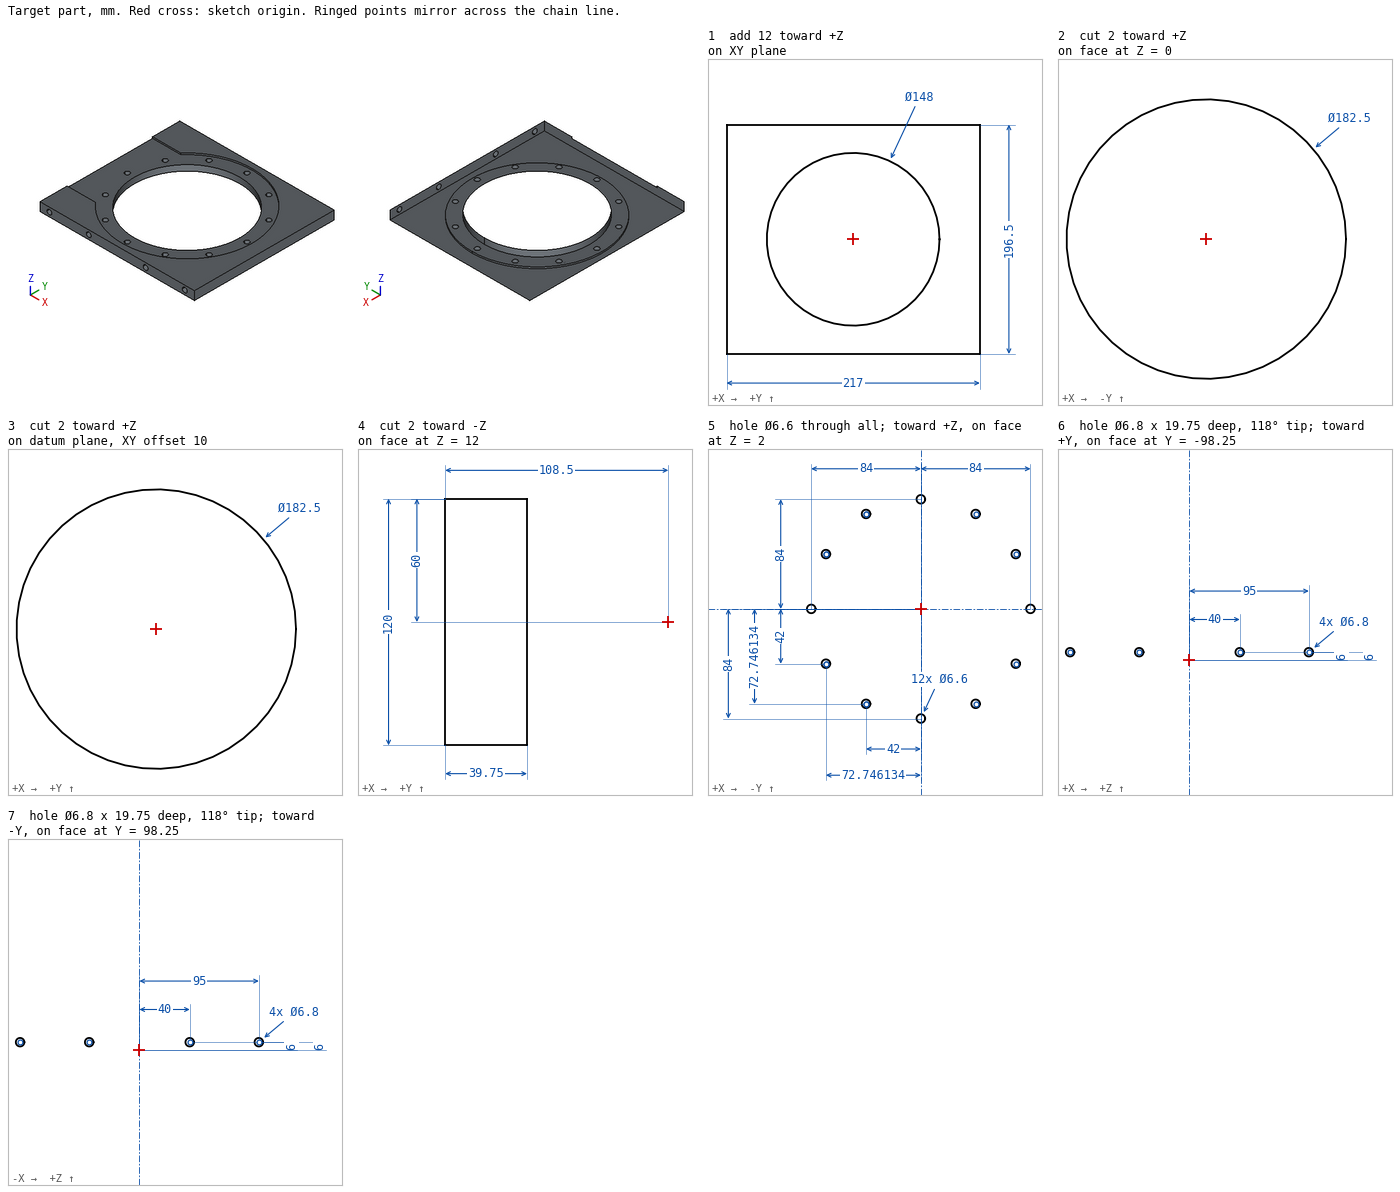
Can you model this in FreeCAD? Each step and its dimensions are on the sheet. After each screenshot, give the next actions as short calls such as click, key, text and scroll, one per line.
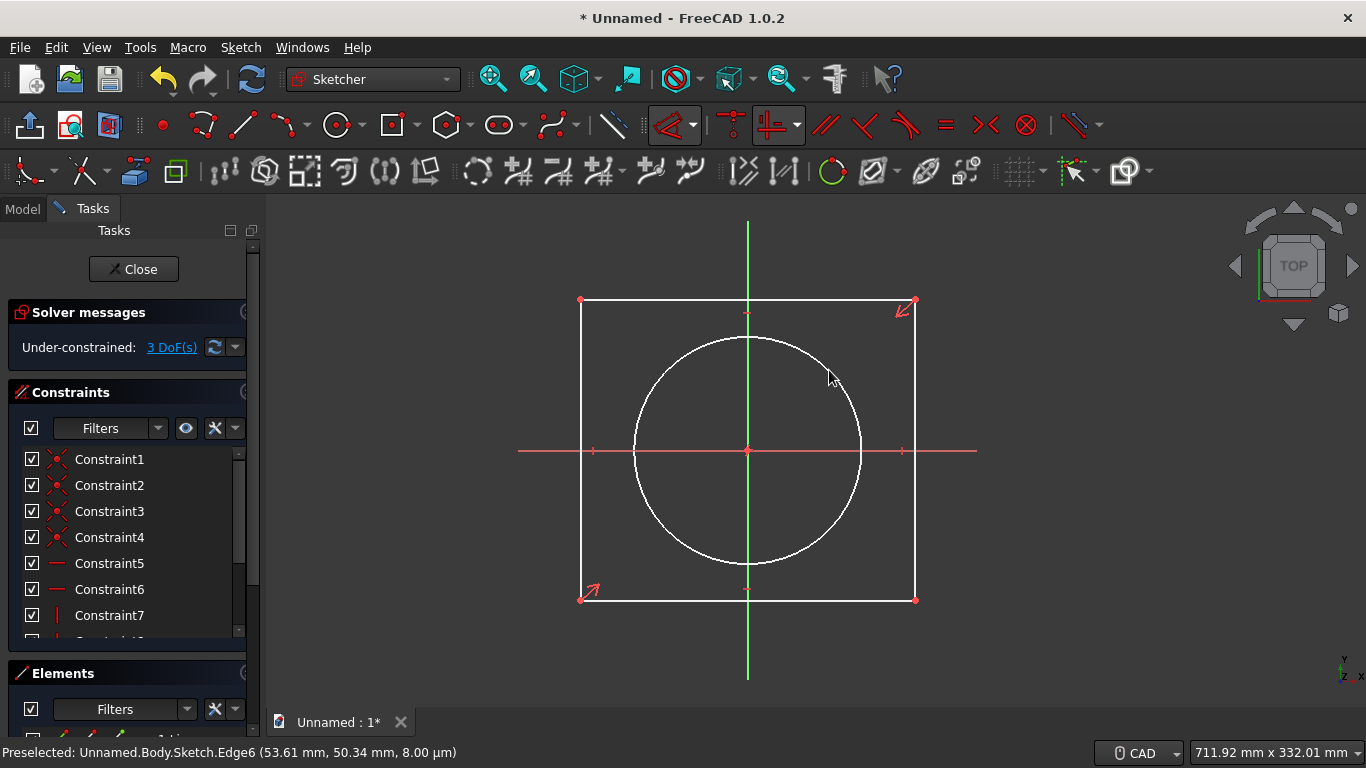
click(668, 126)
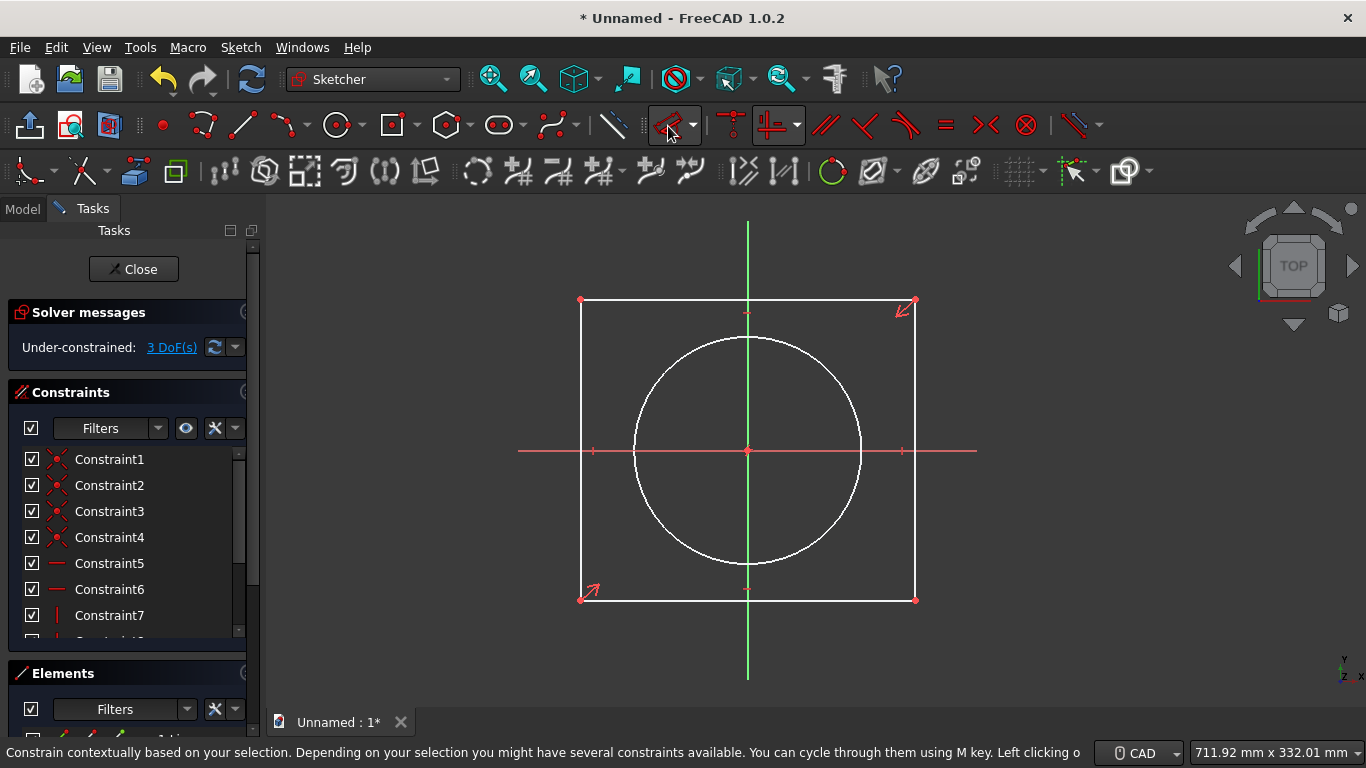
click(828, 370)
click(851, 347)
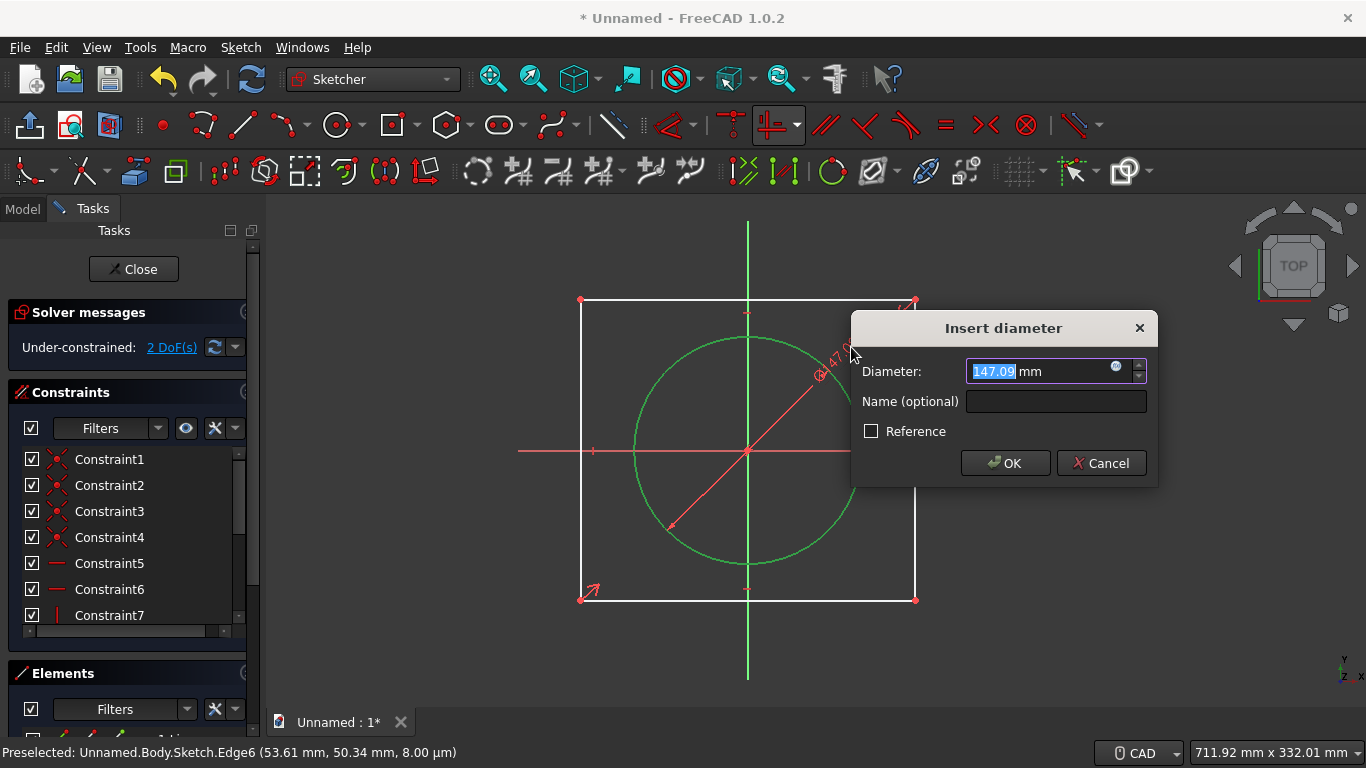
text(148)
key(Return)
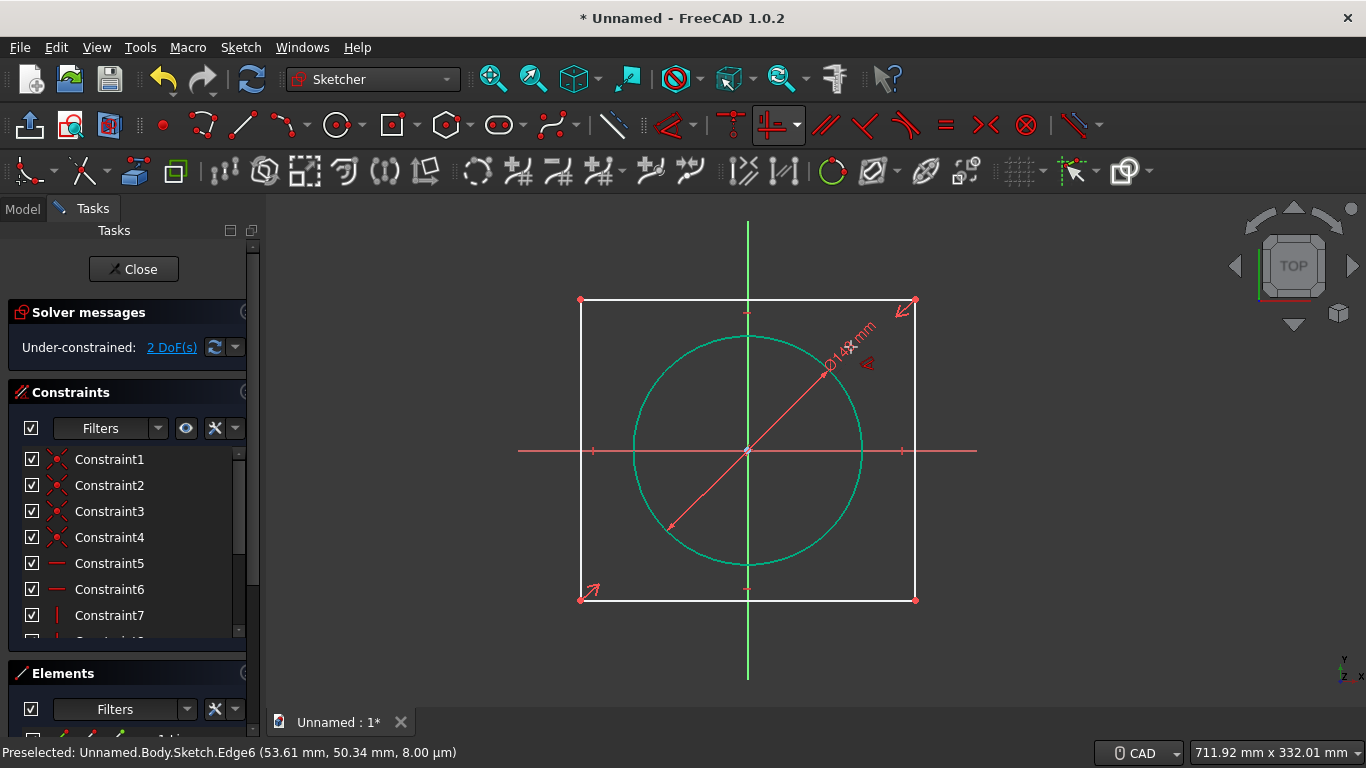
click(681, 601)
click(671, 635)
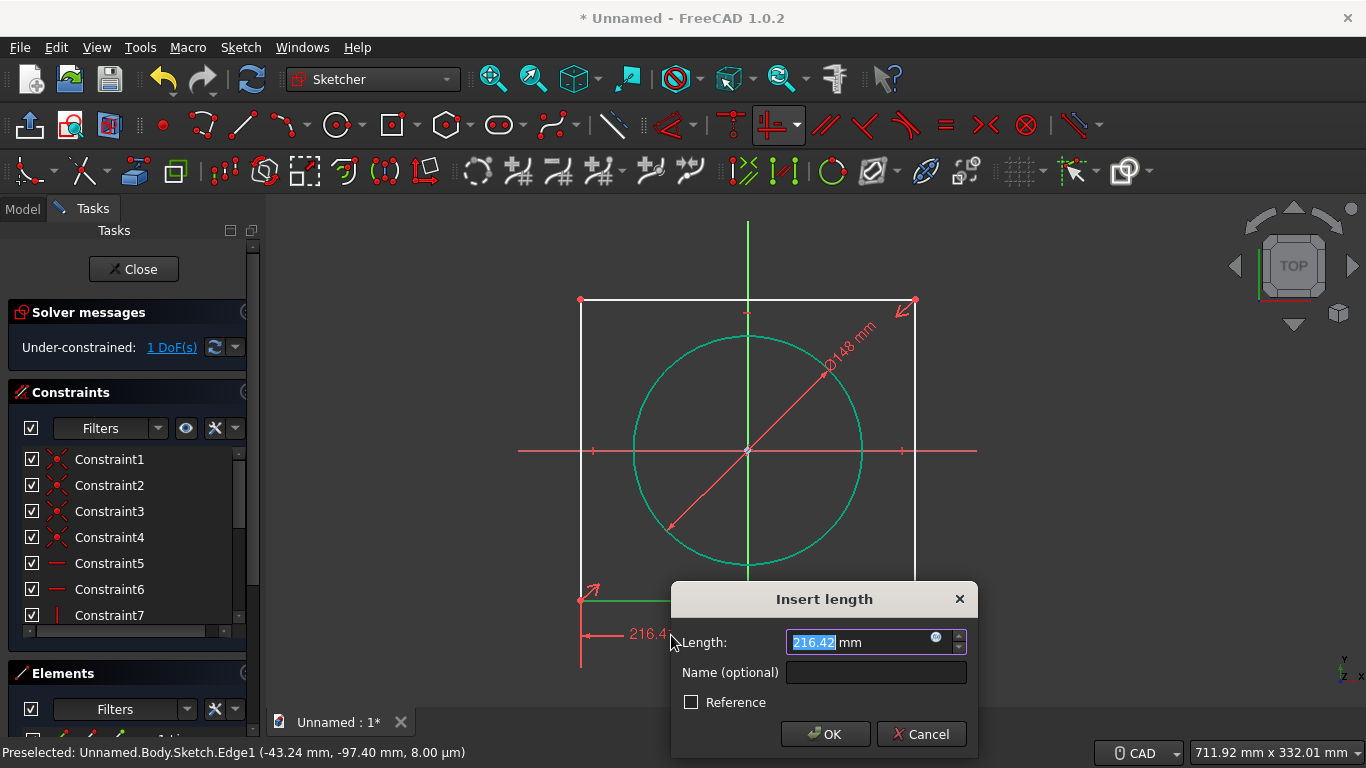
text(217)
key(Return)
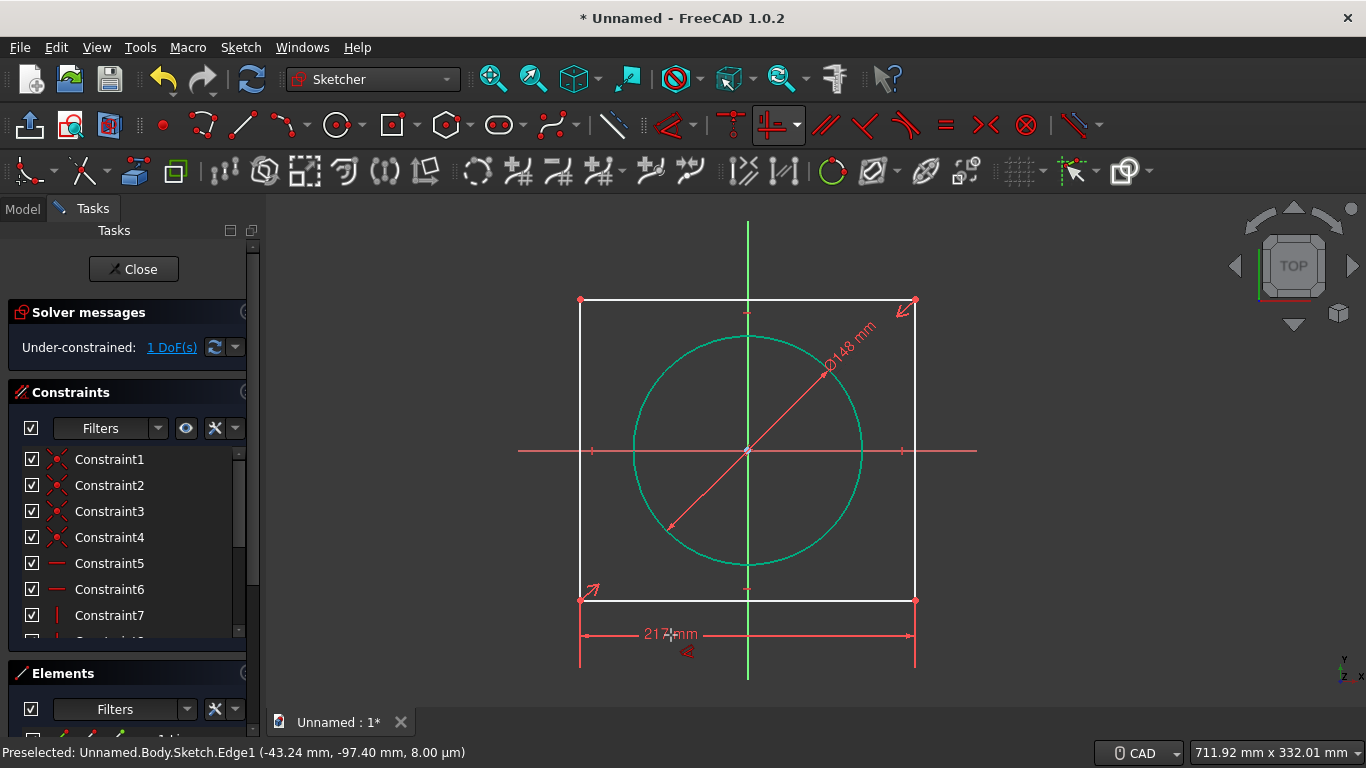
click(915, 511)
click(949, 381)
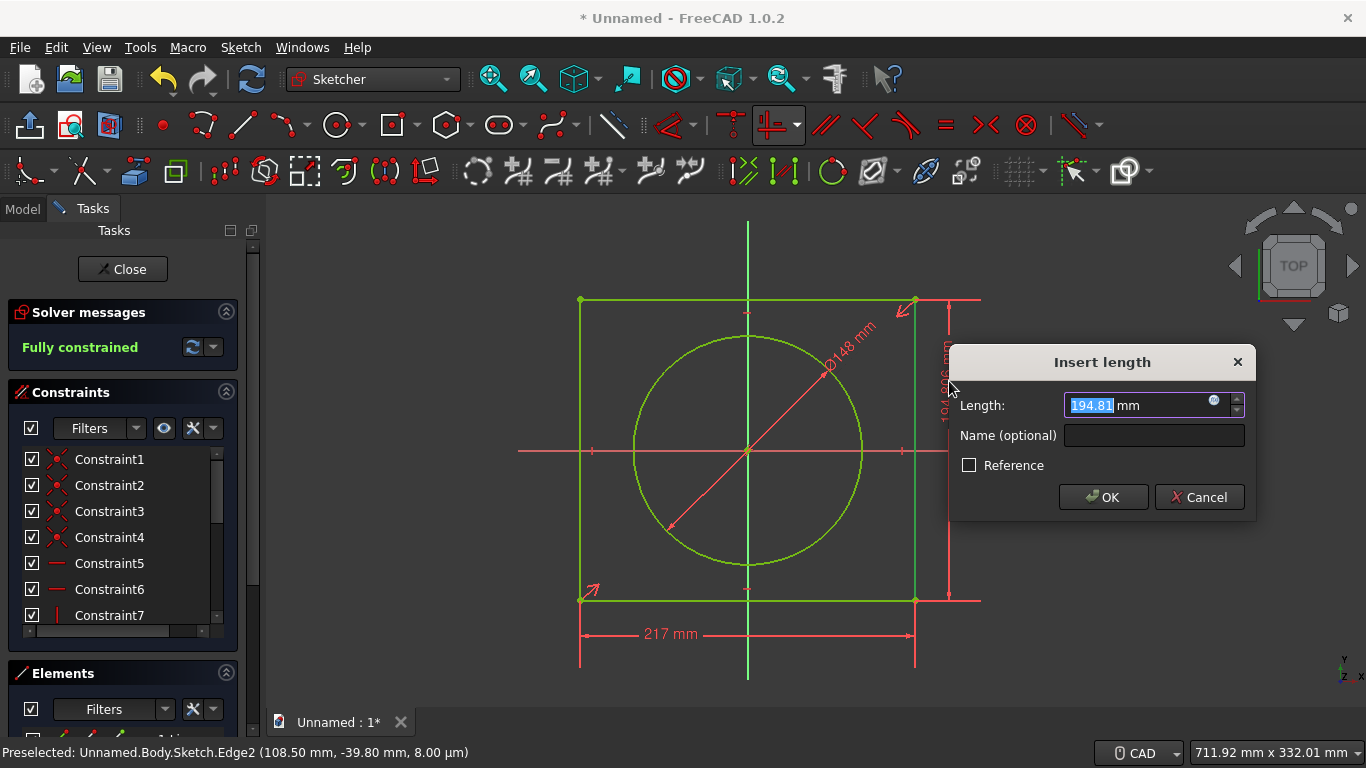
text(196.5)
key(Return)
key(Escape)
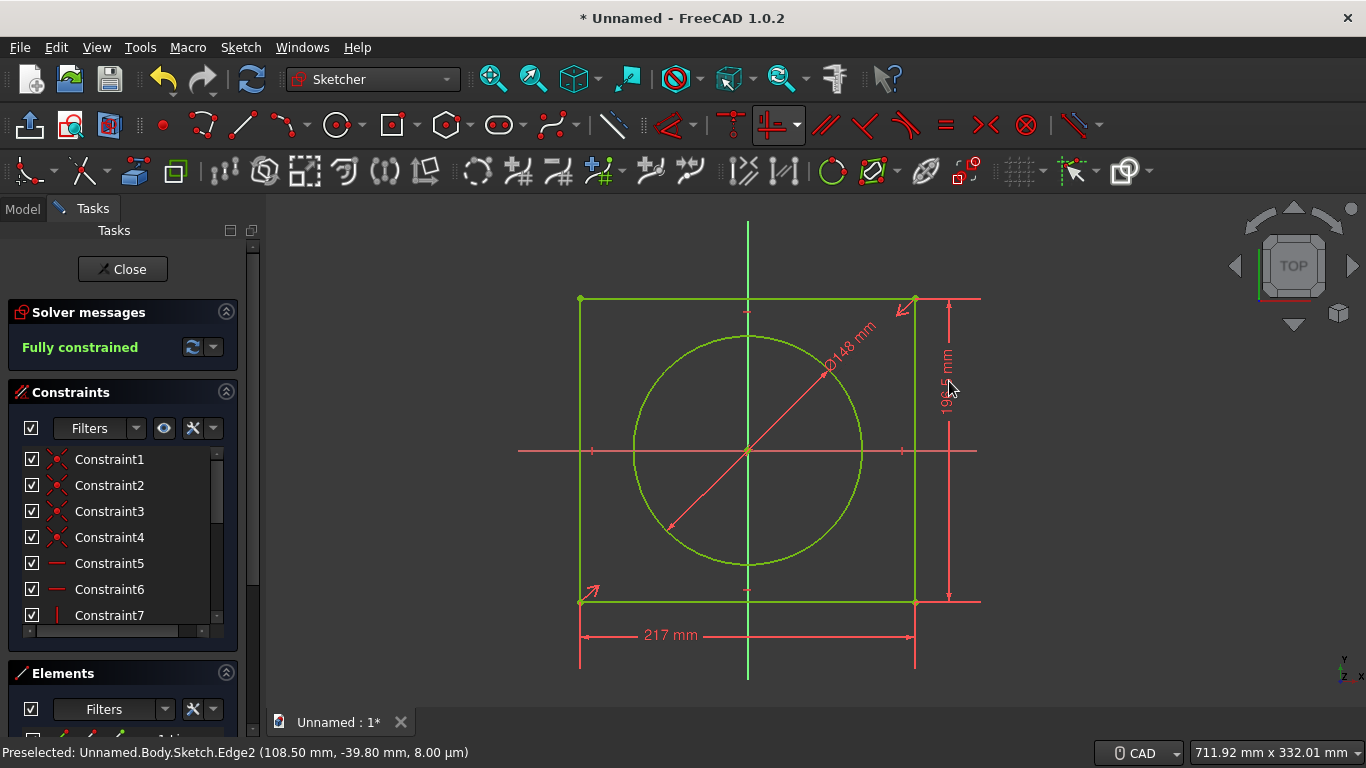
click(123, 269)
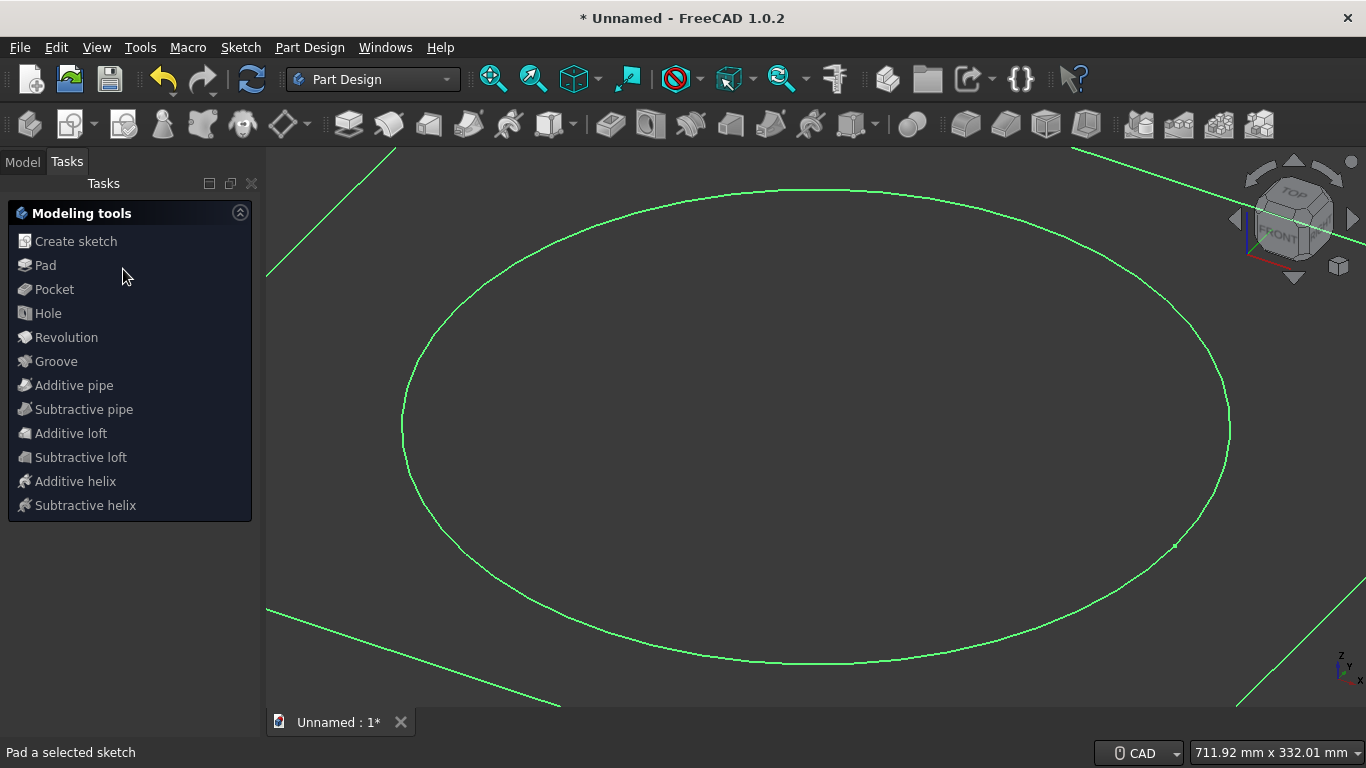
click(350, 124)